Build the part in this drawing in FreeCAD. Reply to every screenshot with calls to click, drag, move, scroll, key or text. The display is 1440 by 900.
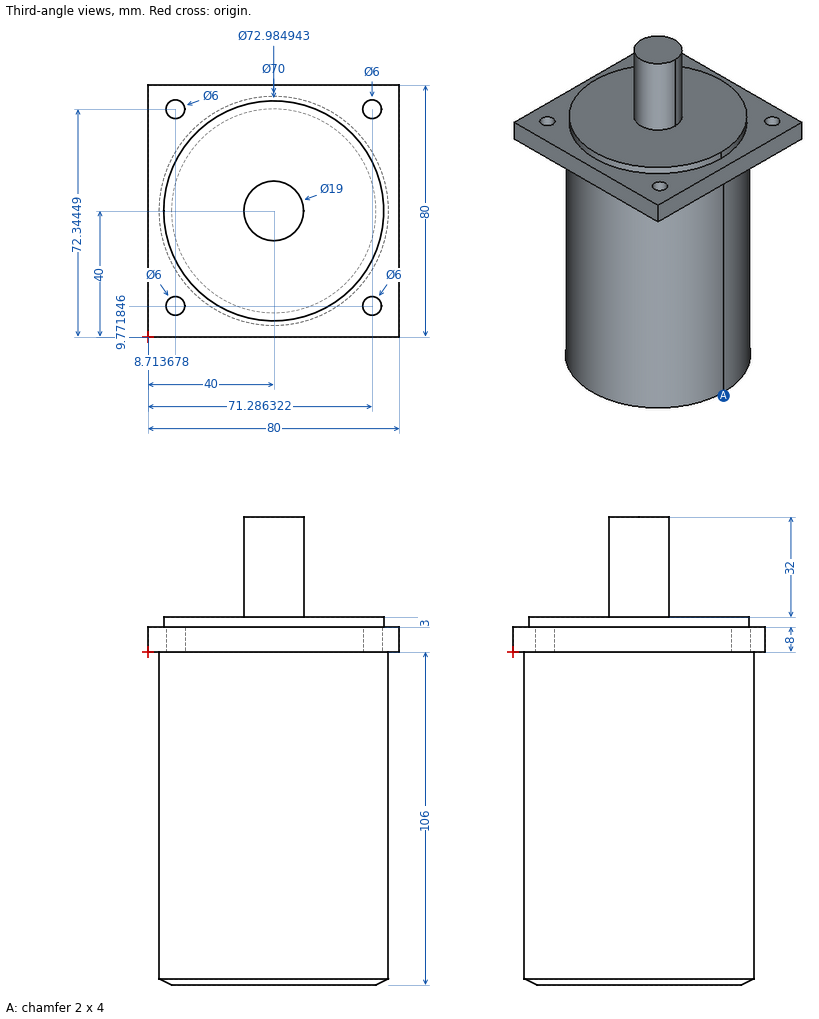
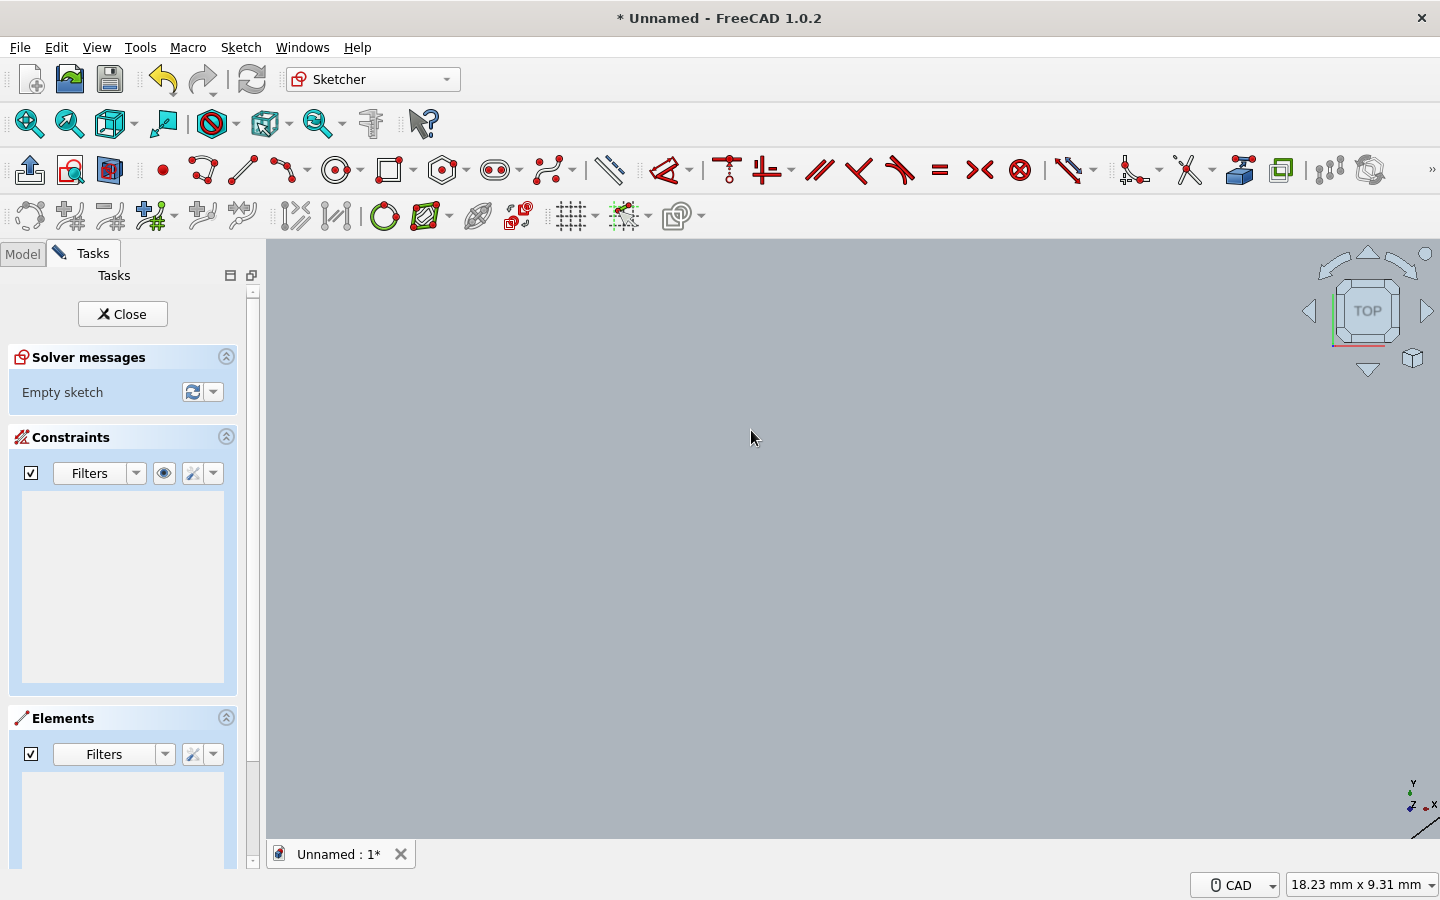
click(336, 170)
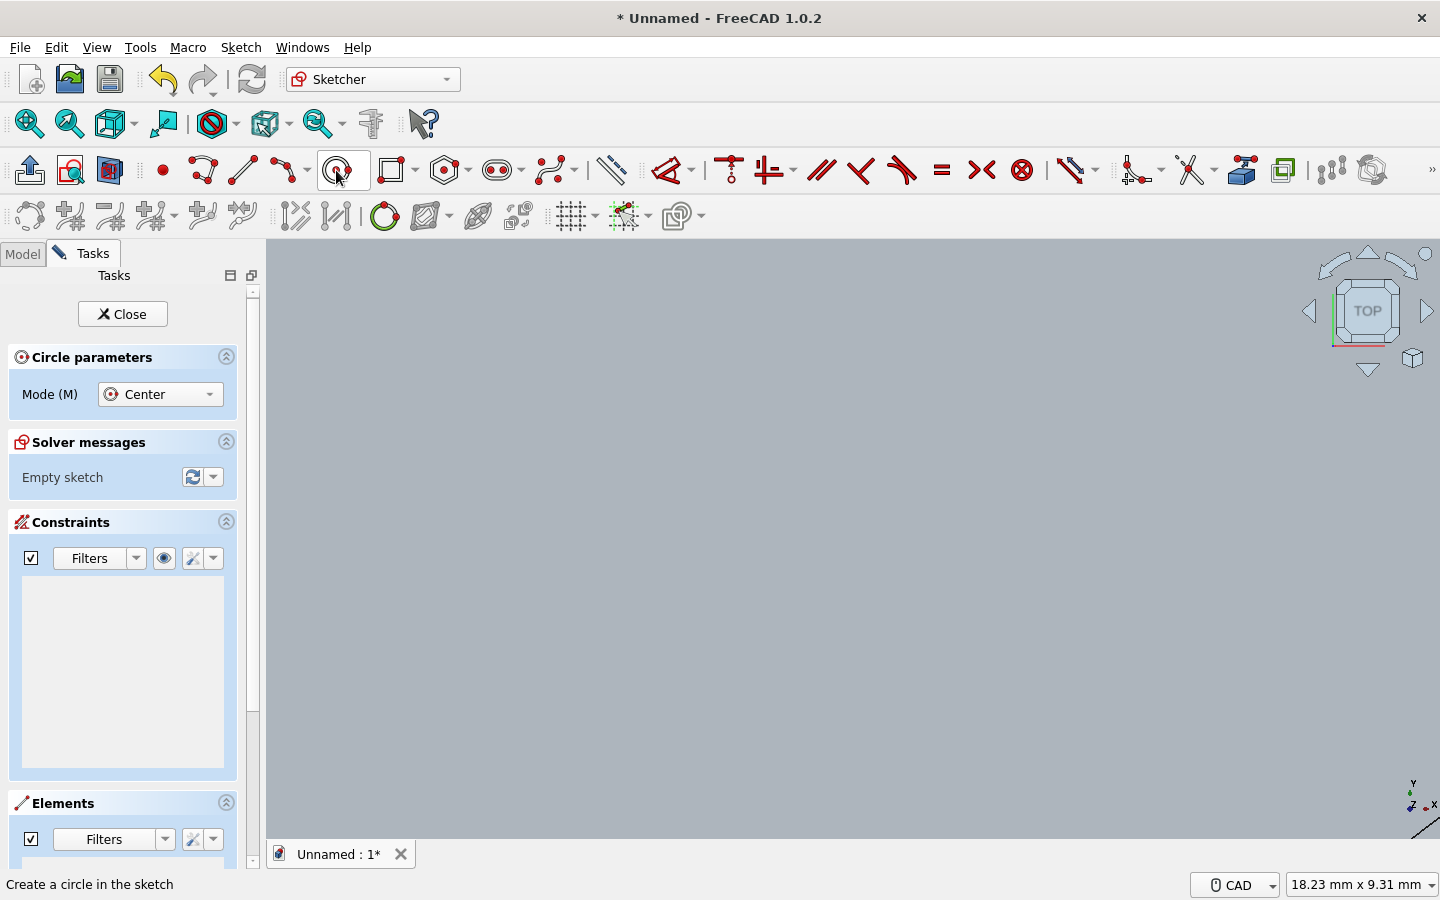
click(776, 530)
move(913, 393)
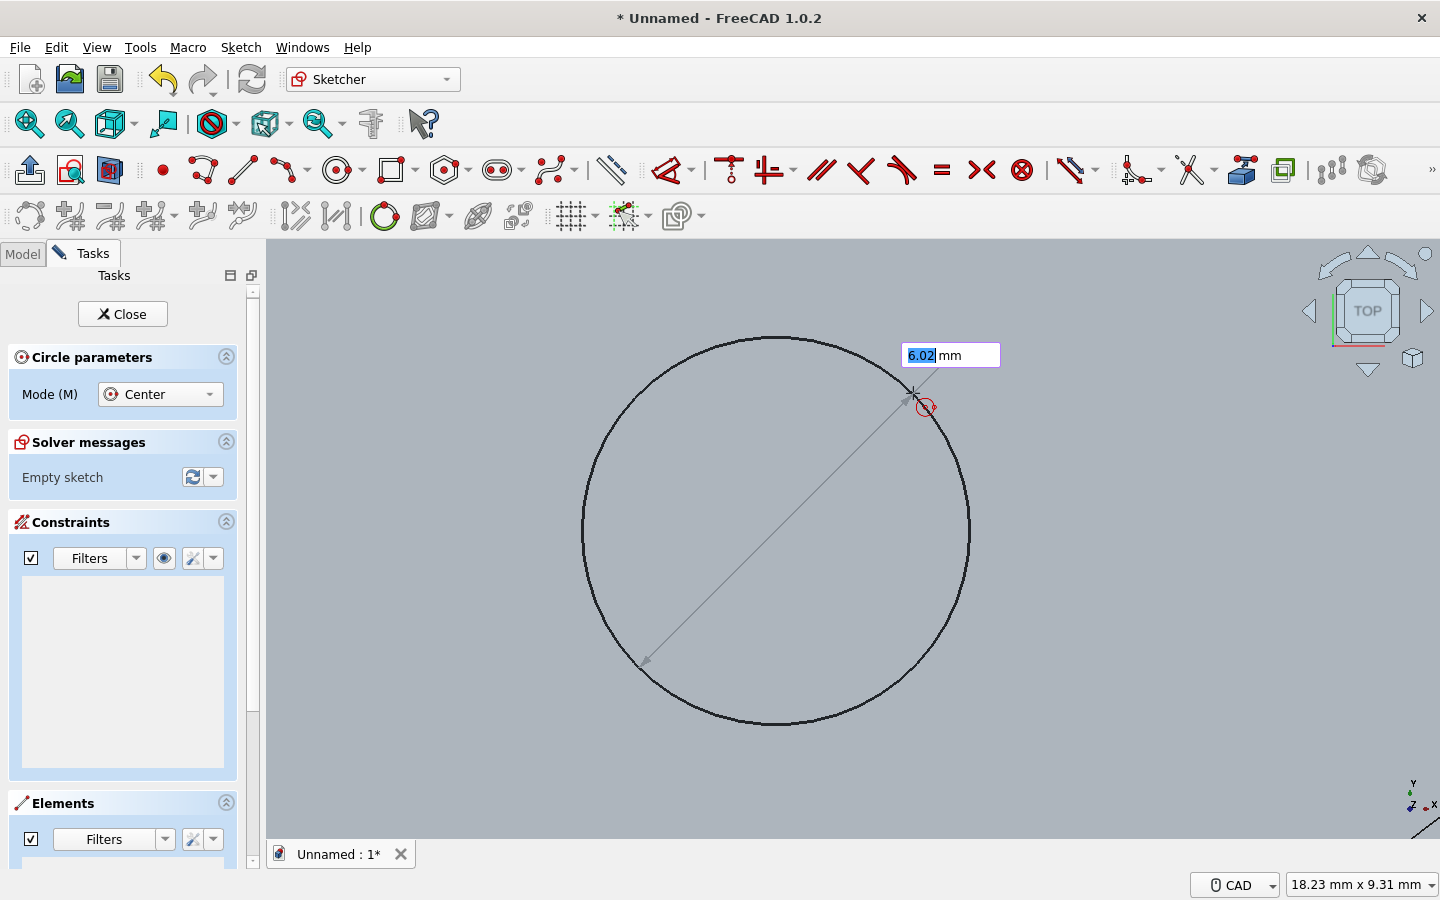
text(6)
key(Return)
key(Escape)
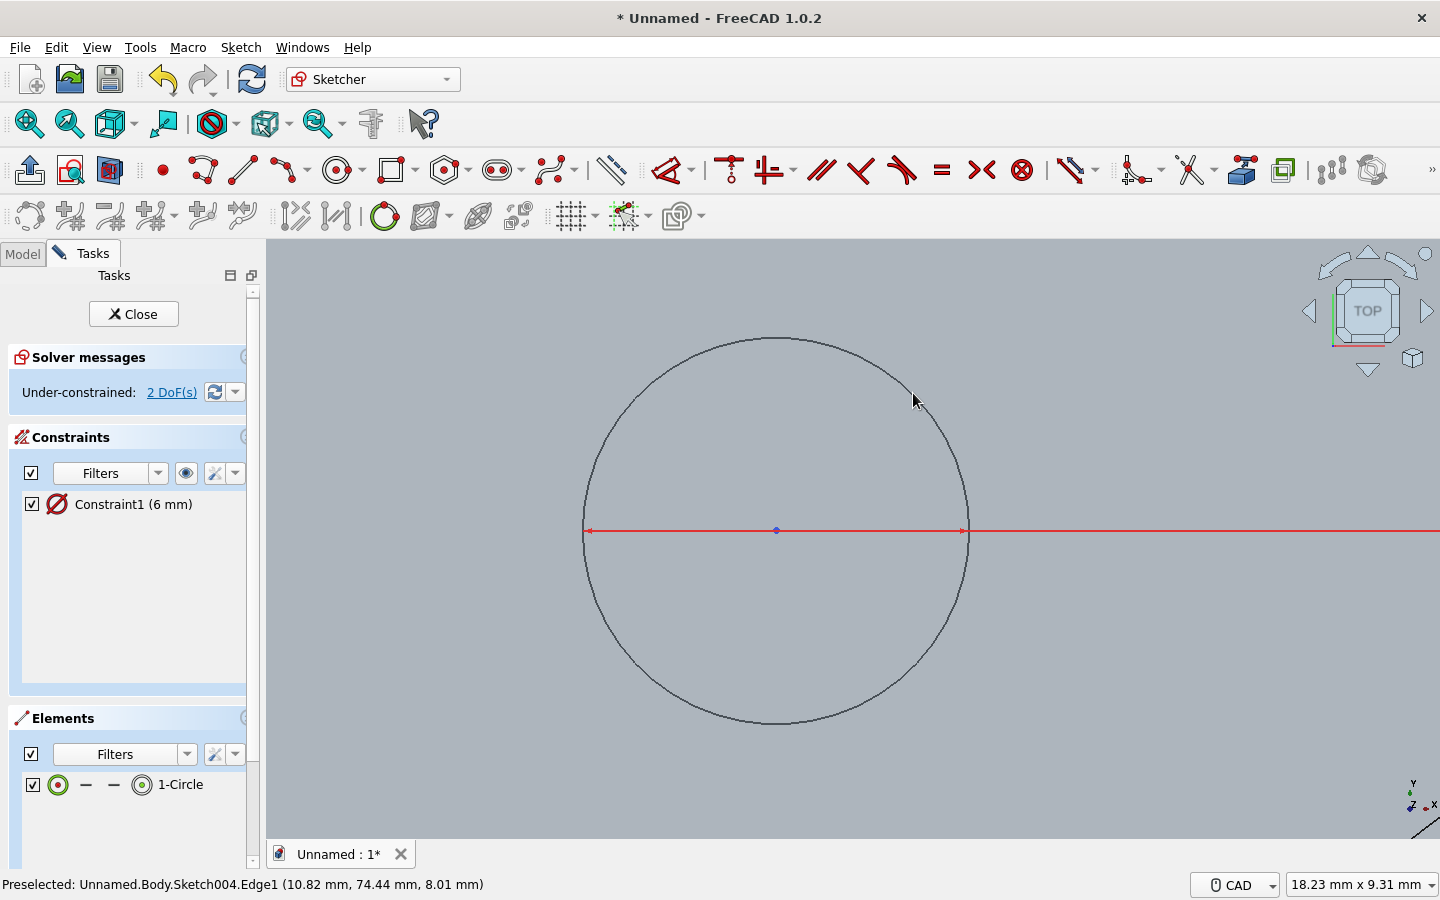
click(666, 170)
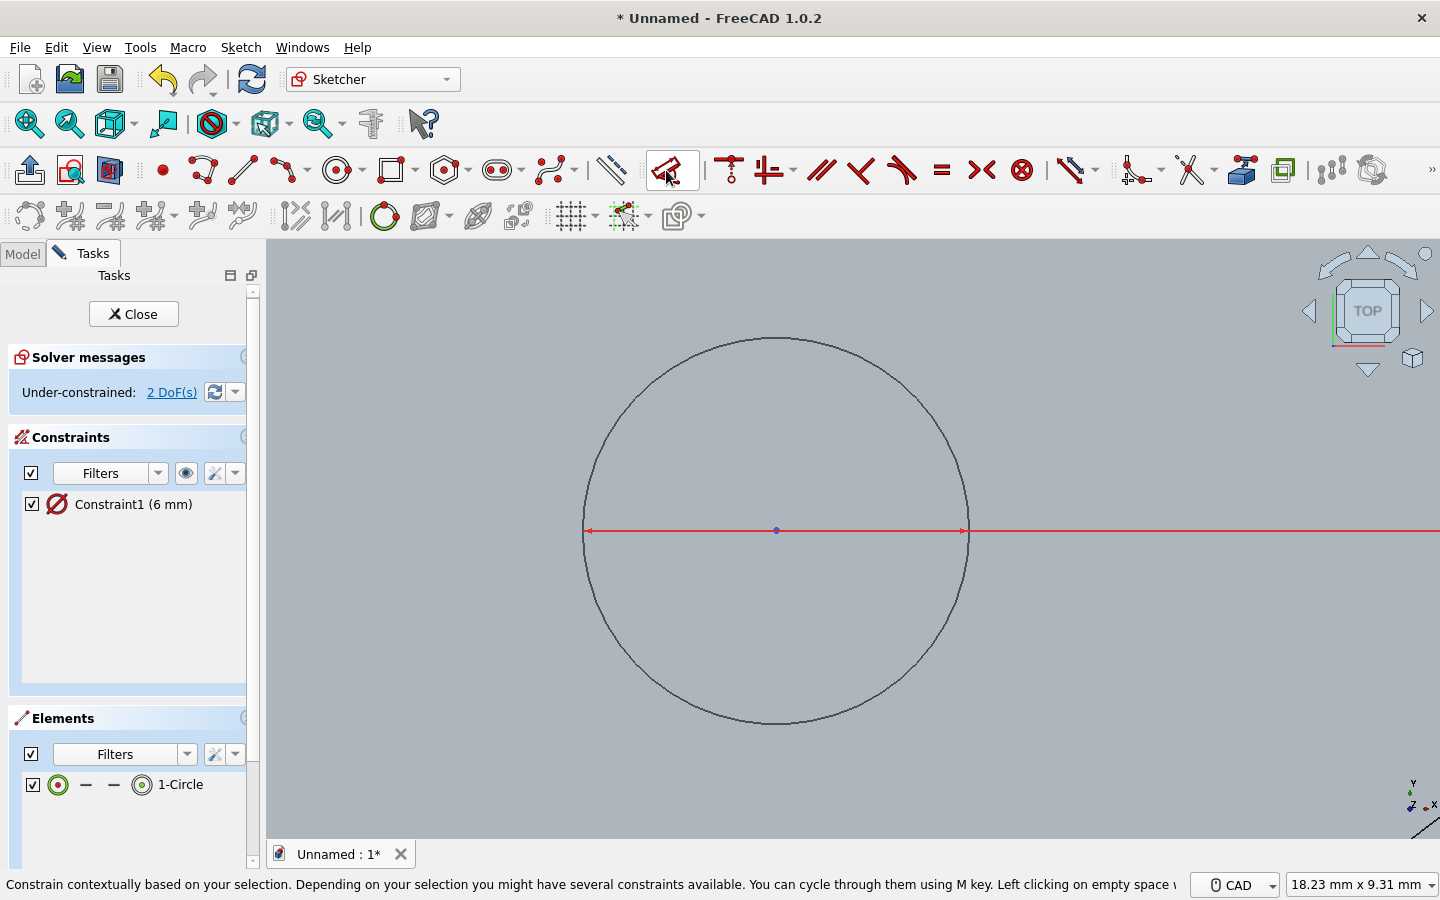
click(776, 531)
click(535, 497)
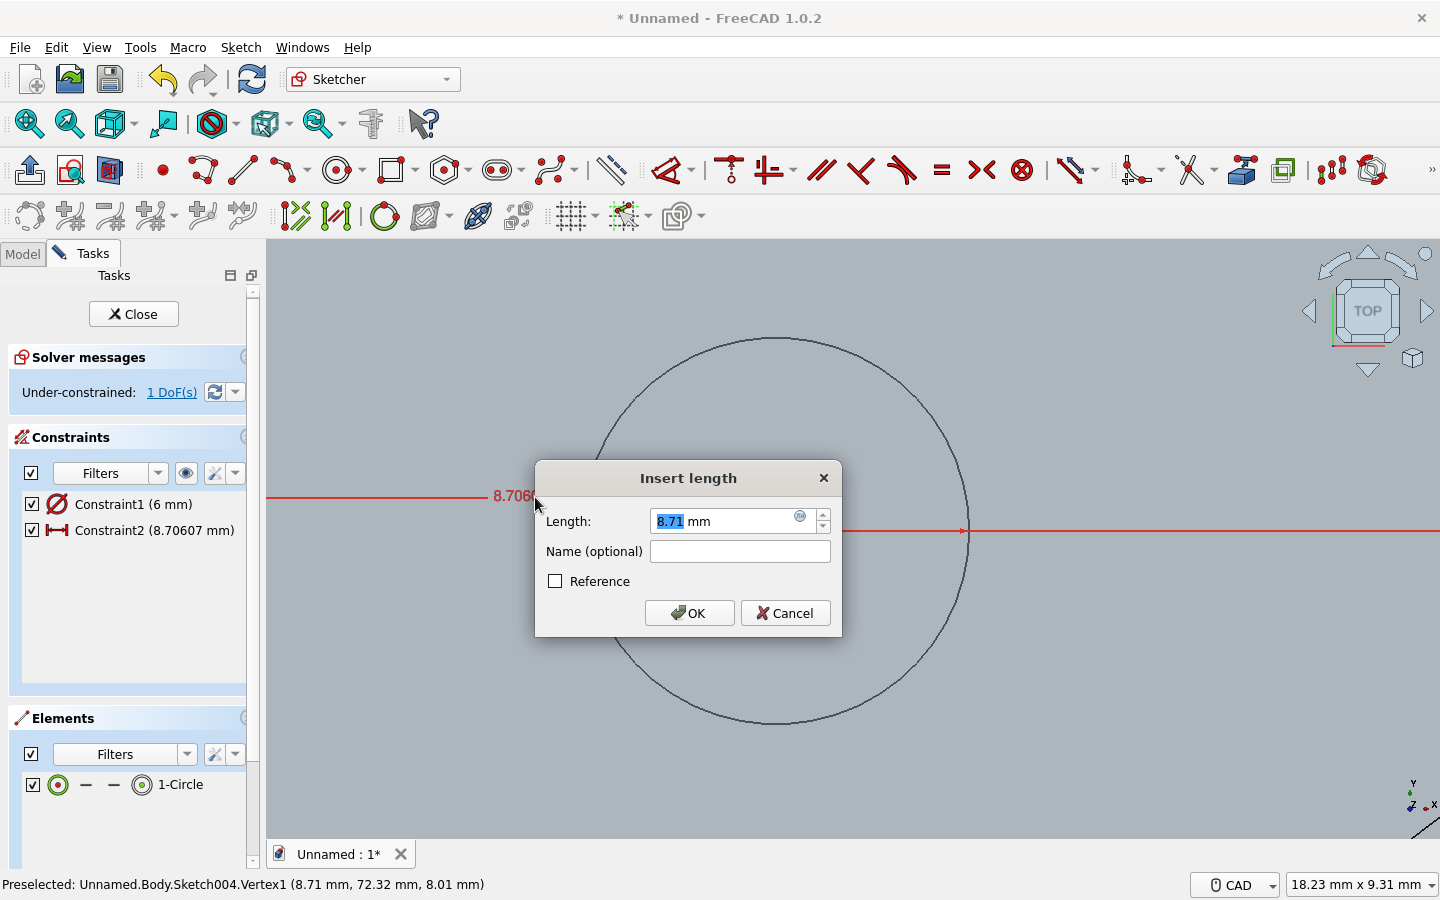
text(8.713678)
key(Return)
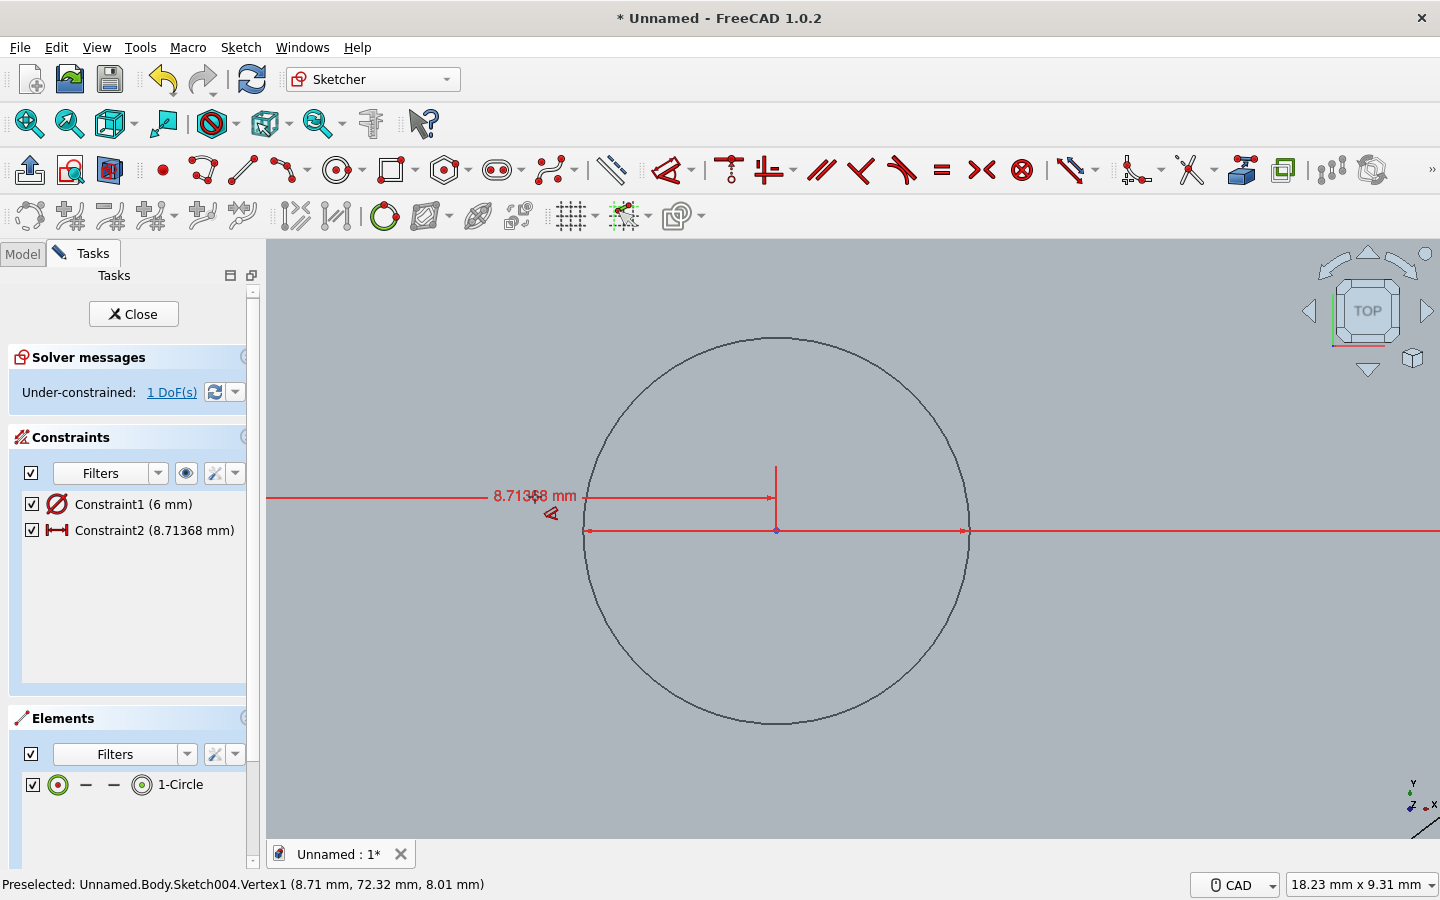
click(776, 531)
click(810, 671)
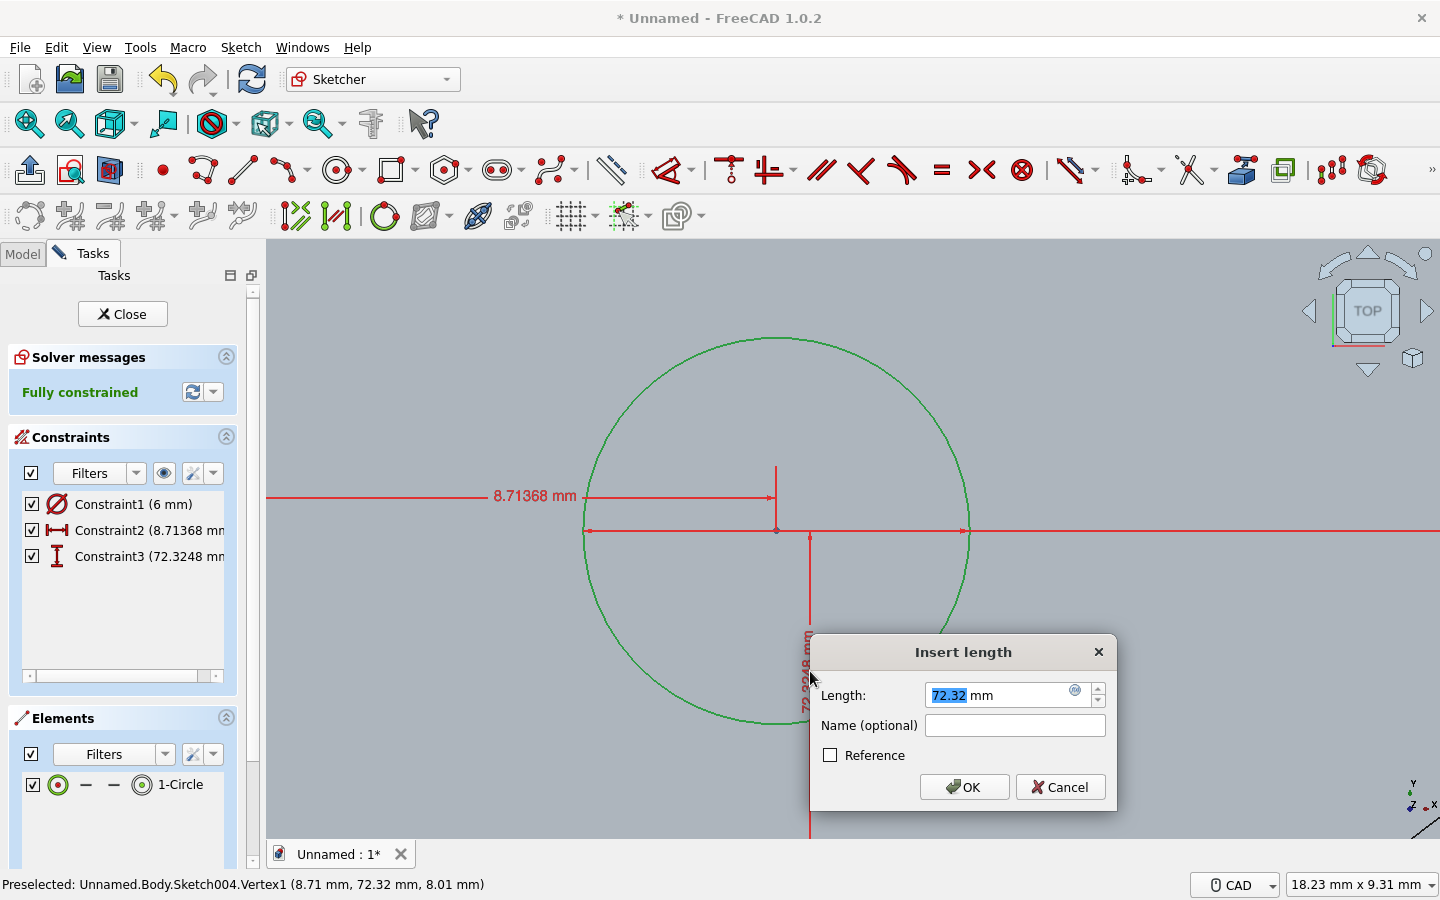
text(72.34449)
key(Return)
key(Escape)